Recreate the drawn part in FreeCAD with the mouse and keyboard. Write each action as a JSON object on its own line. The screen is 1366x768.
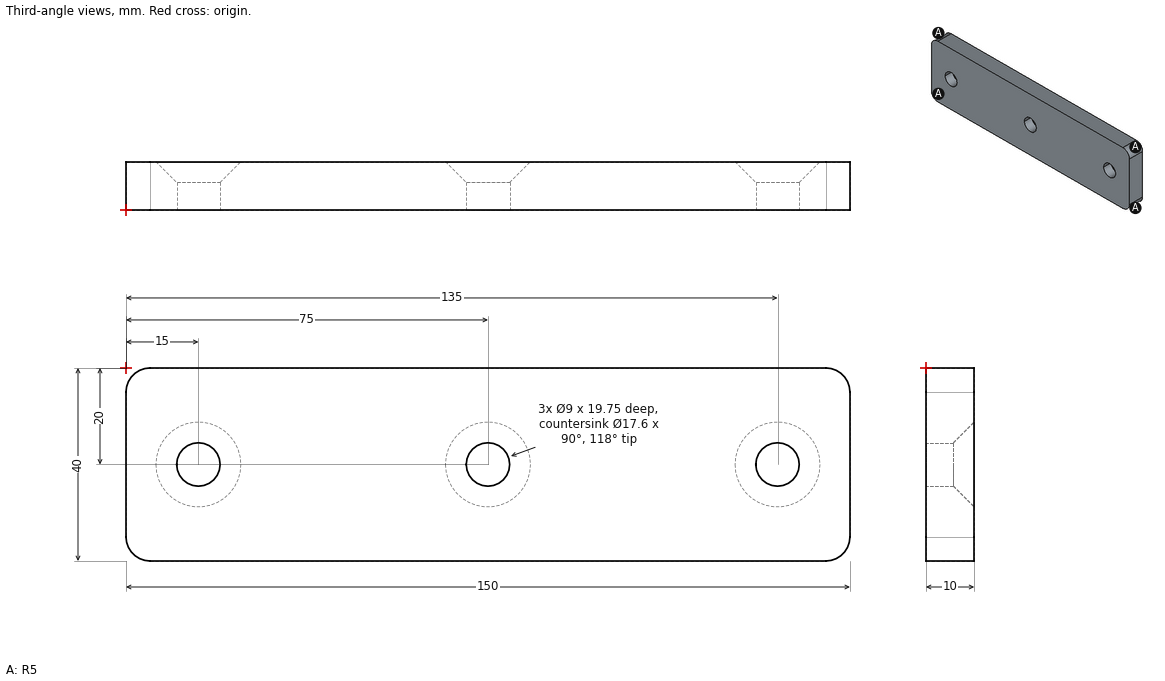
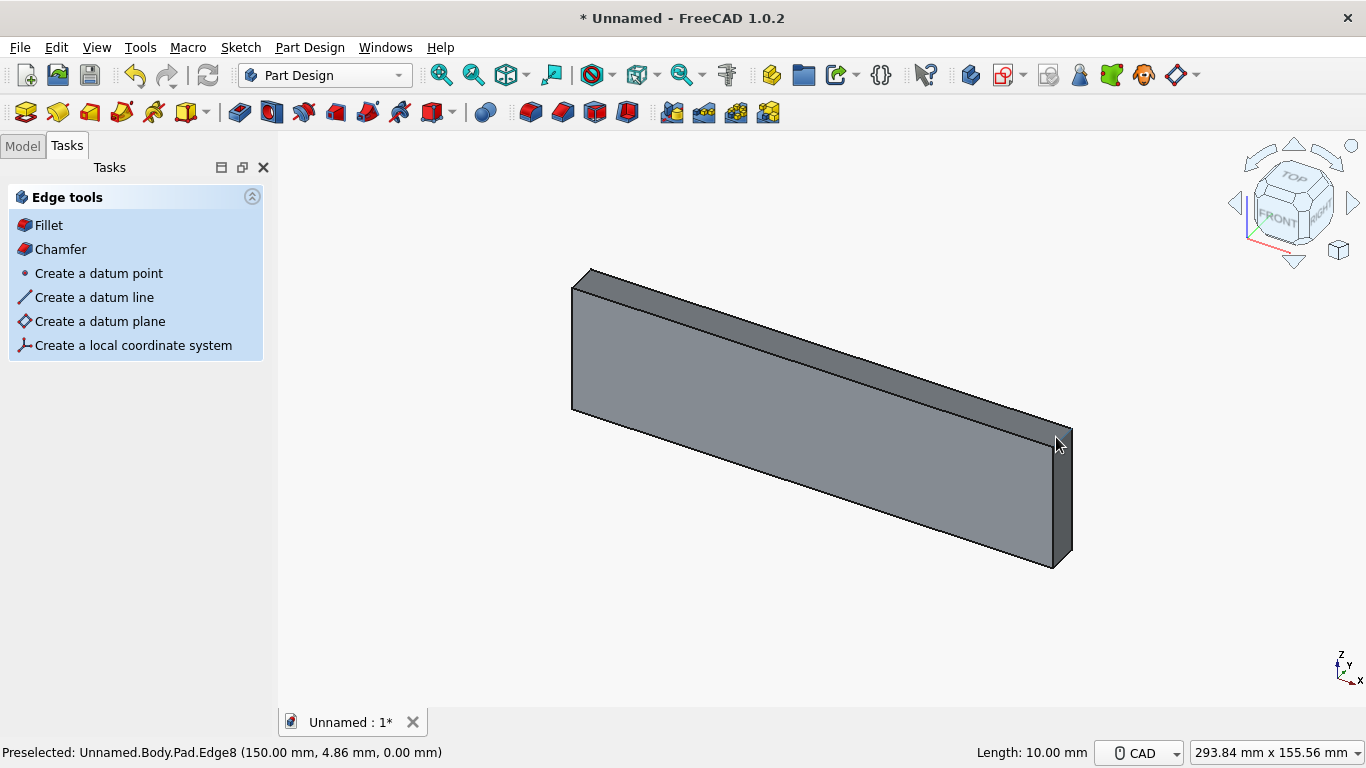
{"action": "key", "text": "0"}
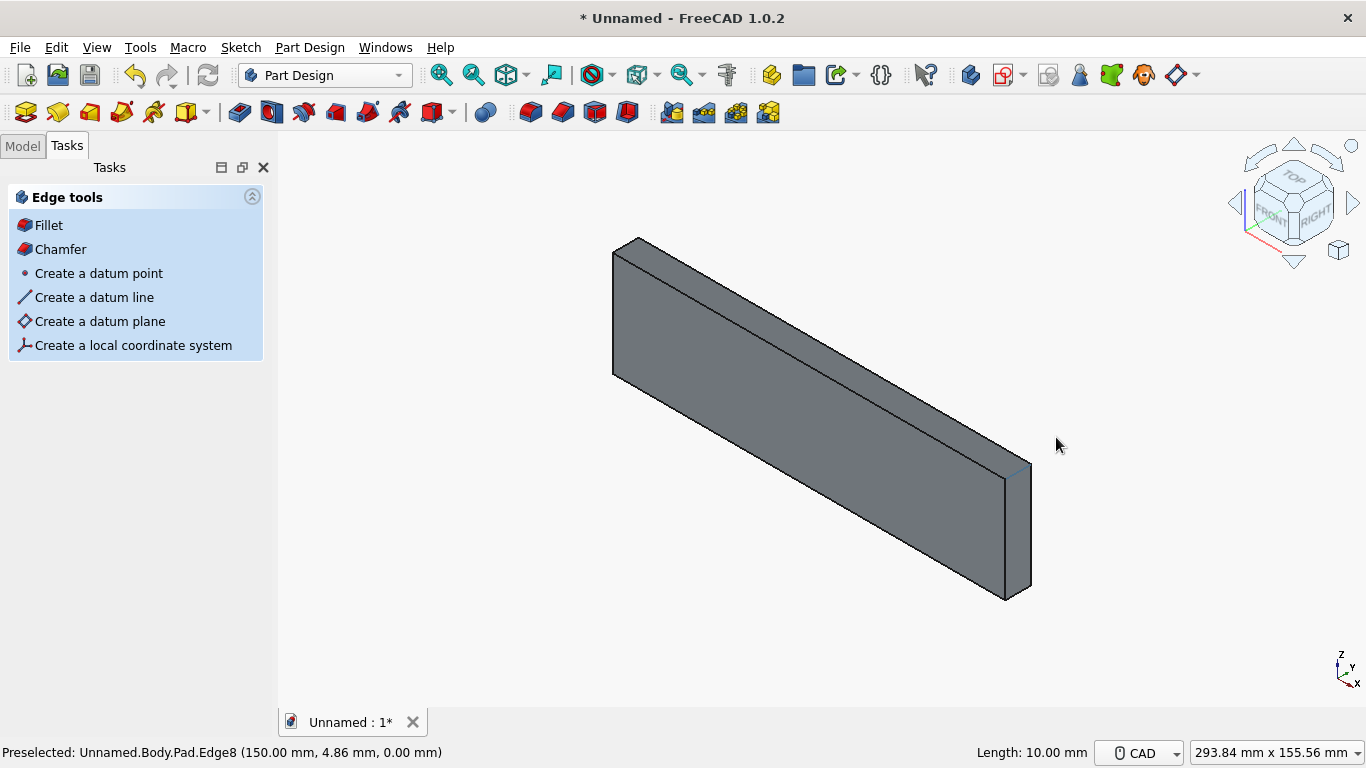
{"action": "key", "text": "2"}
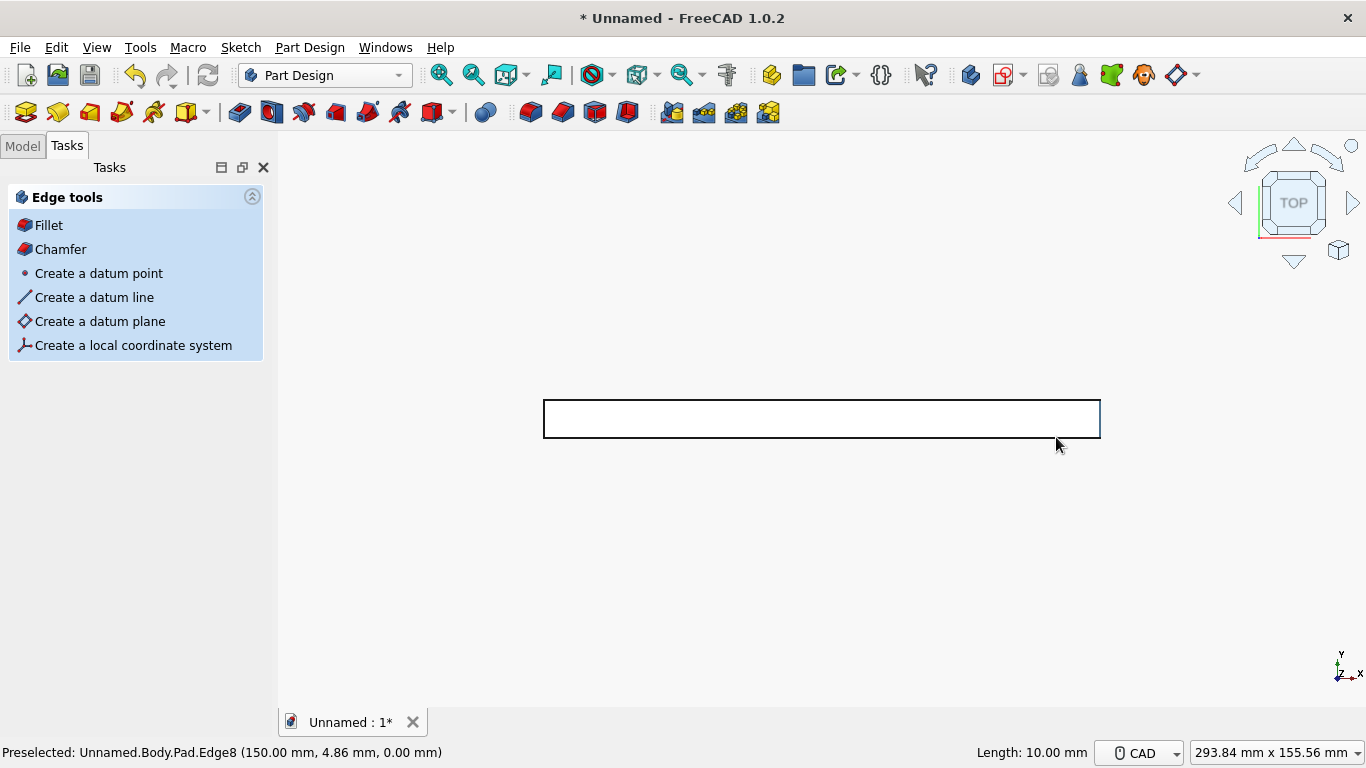
{"action": "left_click", "coordinate": [544, 418], "text": "ctrl"}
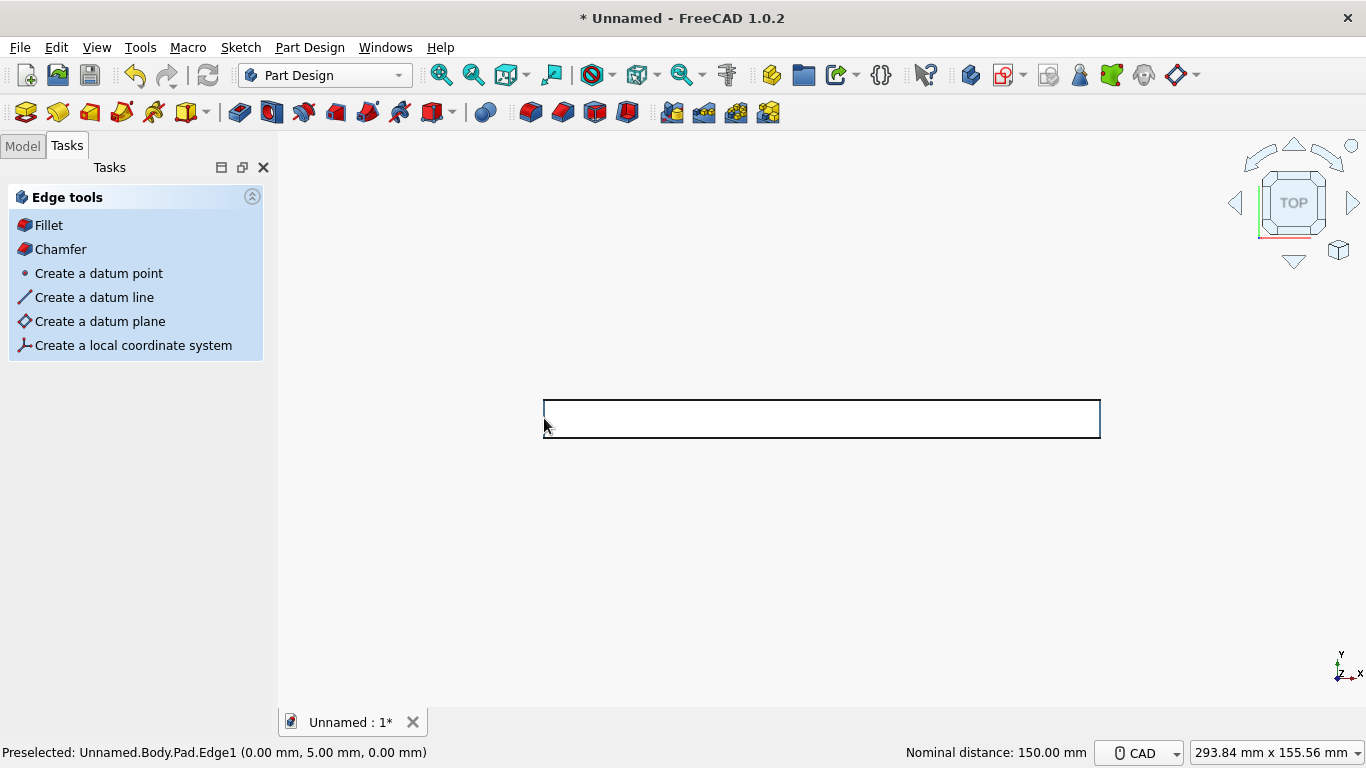
{"action": "key", "text": "1"}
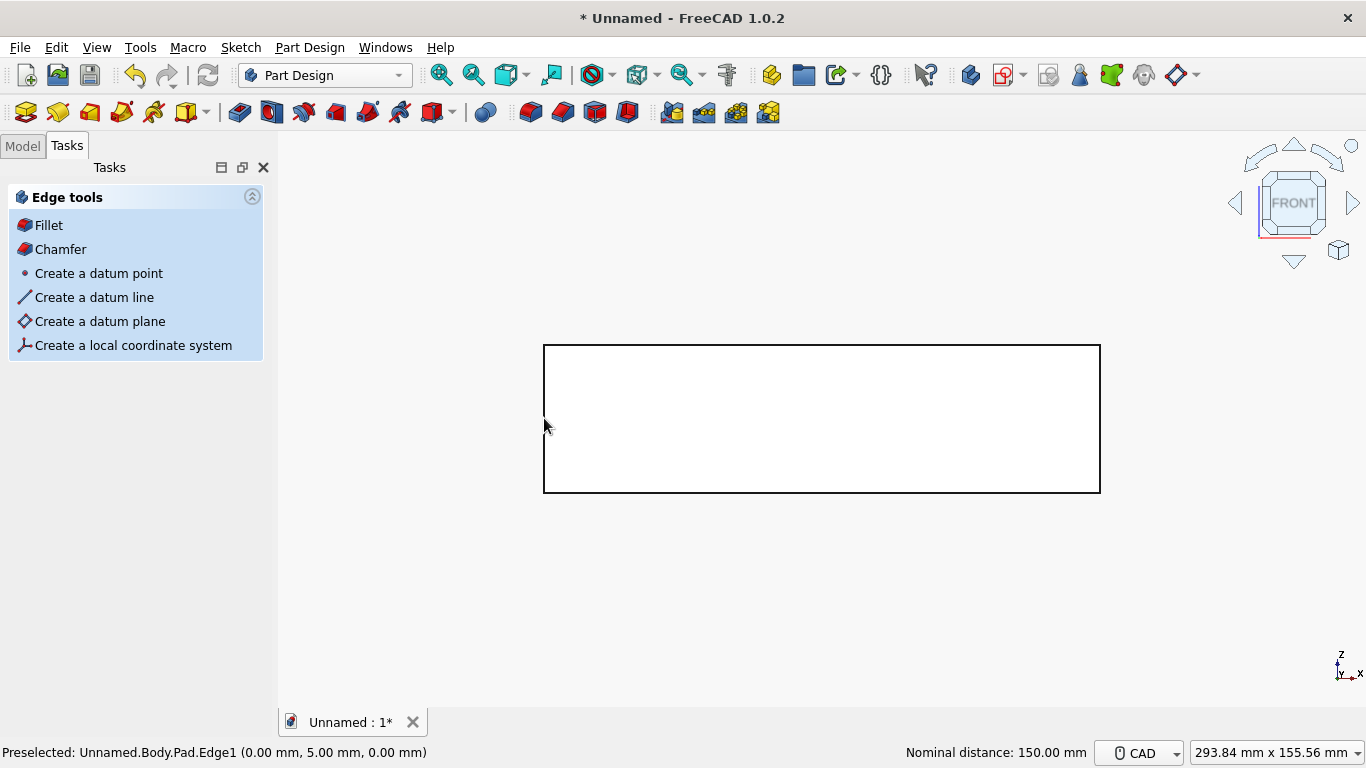
{"action": "key", "text": "3"}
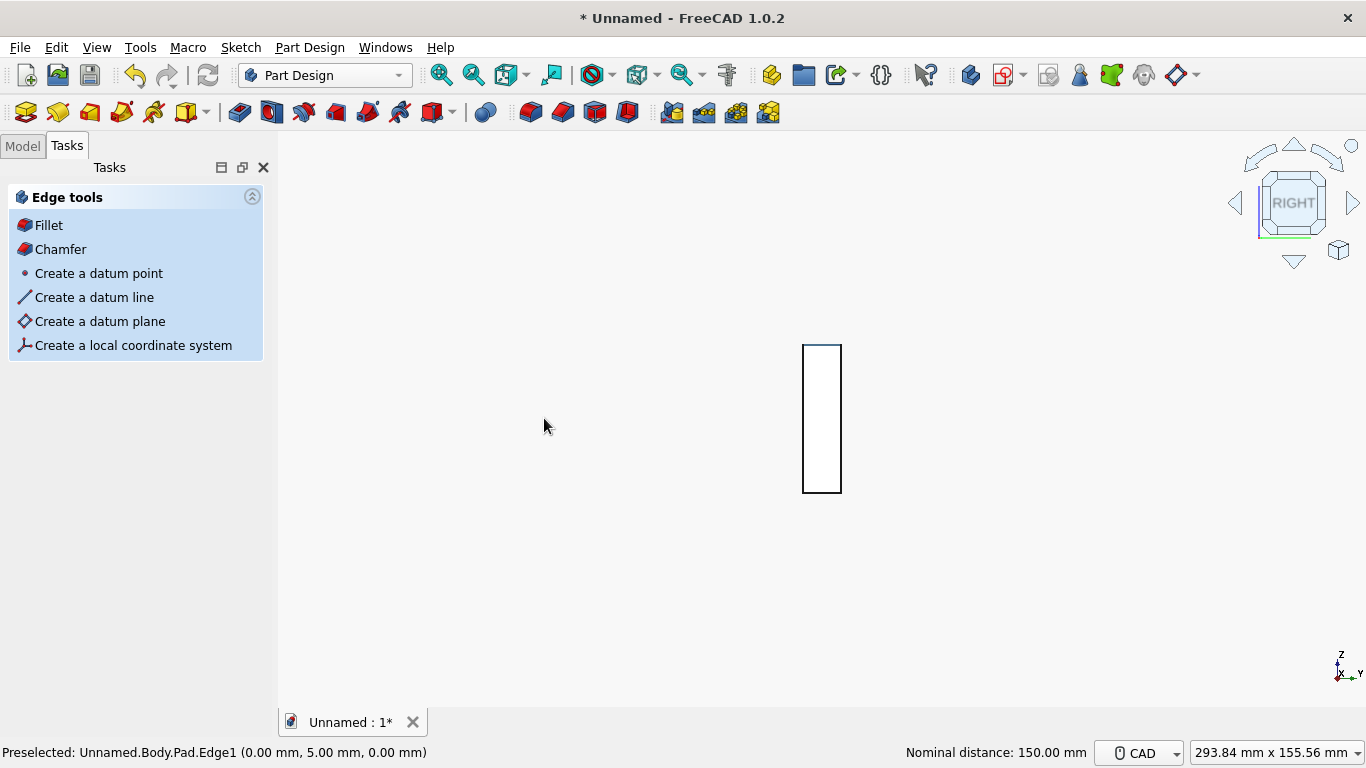
{"action": "left_click", "coordinate": [442, 76]}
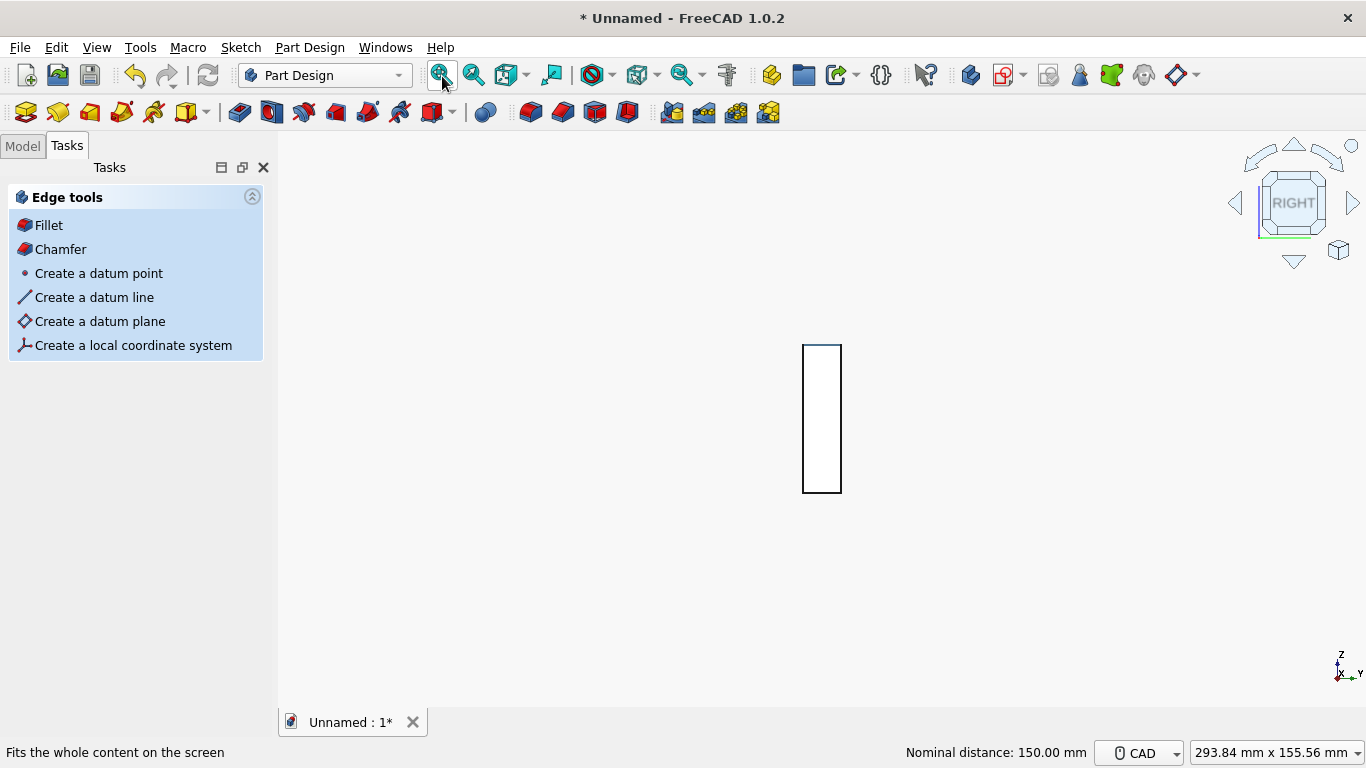
{"action": "left_click", "coordinate": [822, 492], "text": "ctrl"}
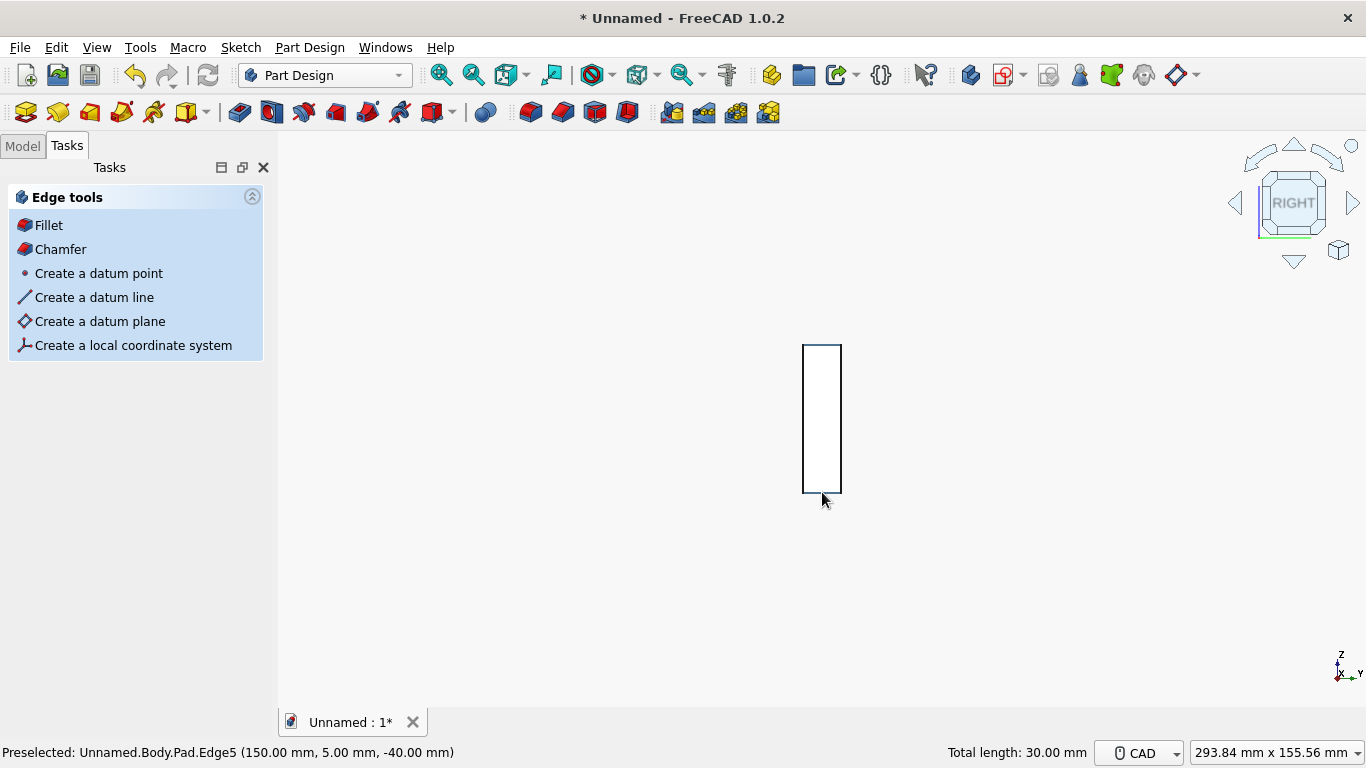
{"action": "key", "text": "5"}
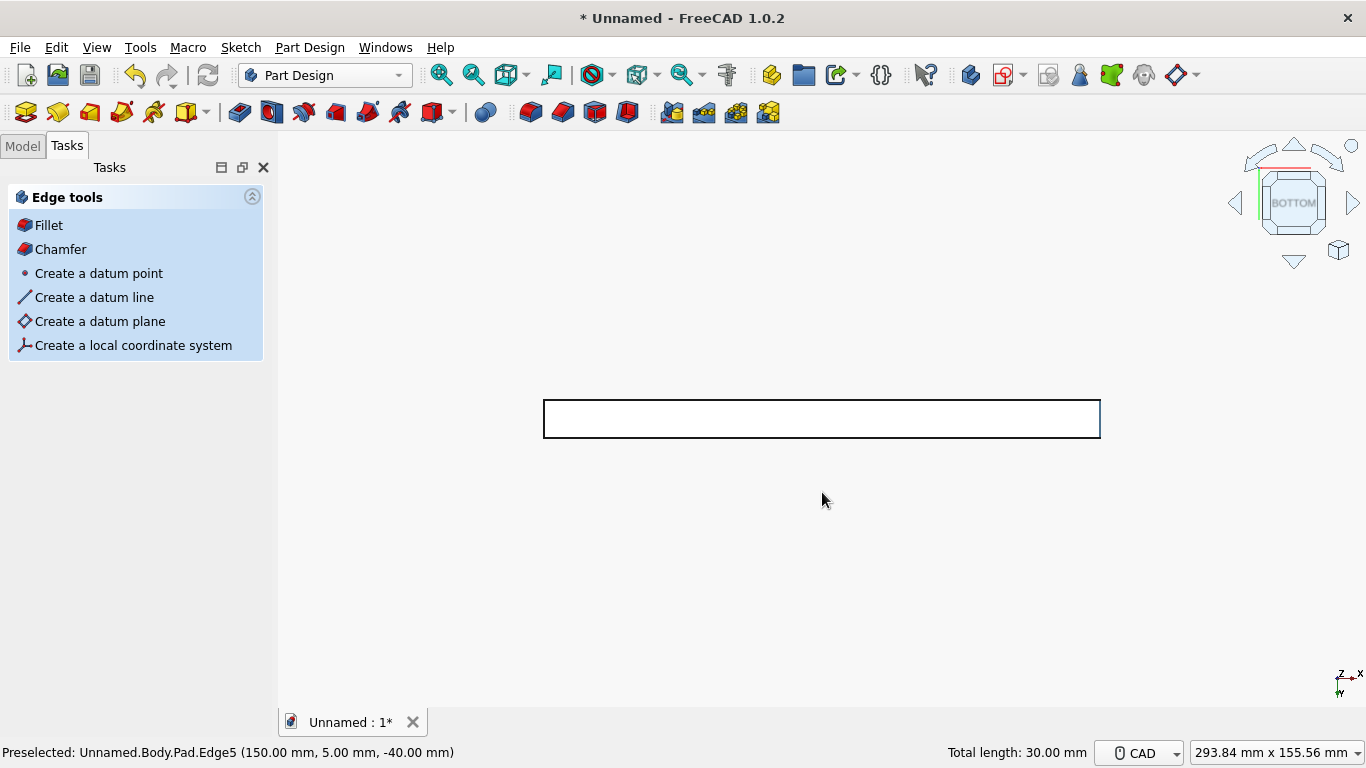
{"action": "left_click", "coordinate": [544, 418], "text": "ctrl"}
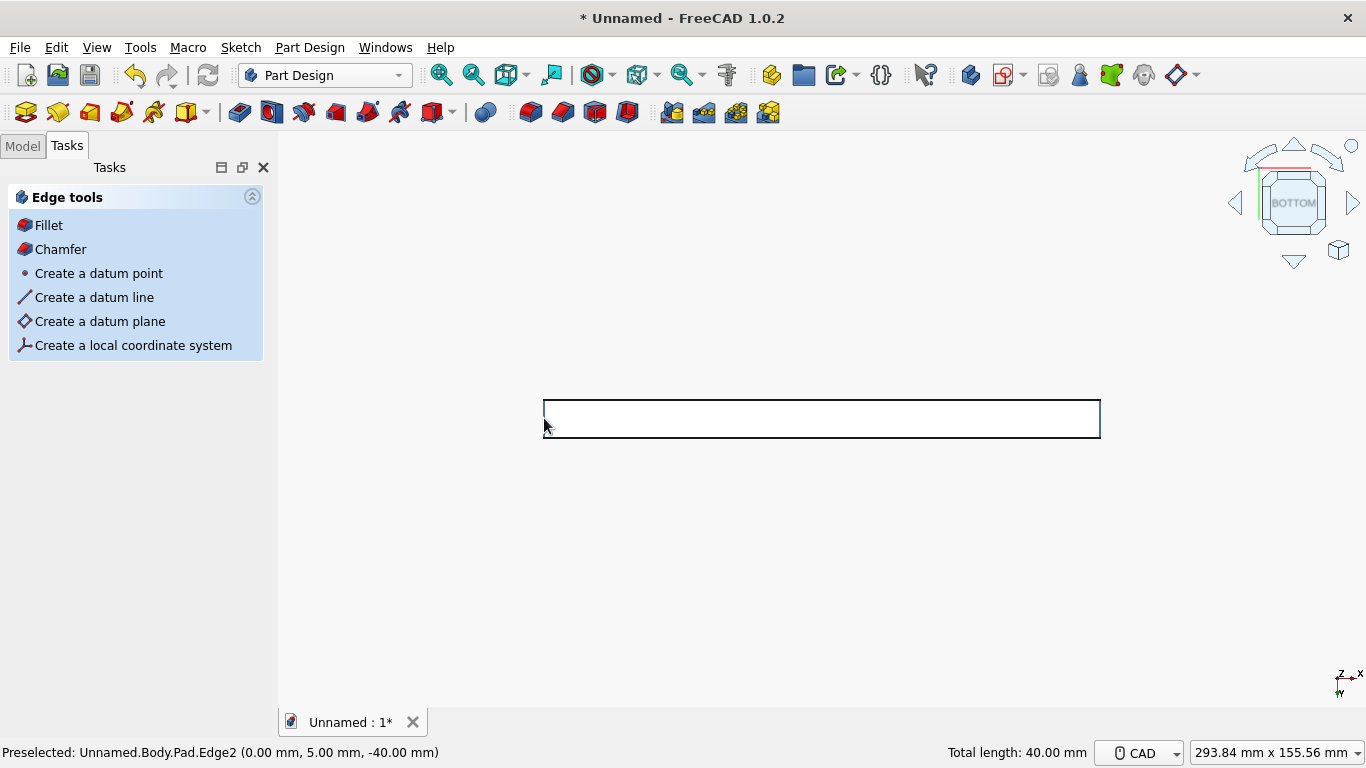
{"action": "left_click", "coordinate": [532, 112]}